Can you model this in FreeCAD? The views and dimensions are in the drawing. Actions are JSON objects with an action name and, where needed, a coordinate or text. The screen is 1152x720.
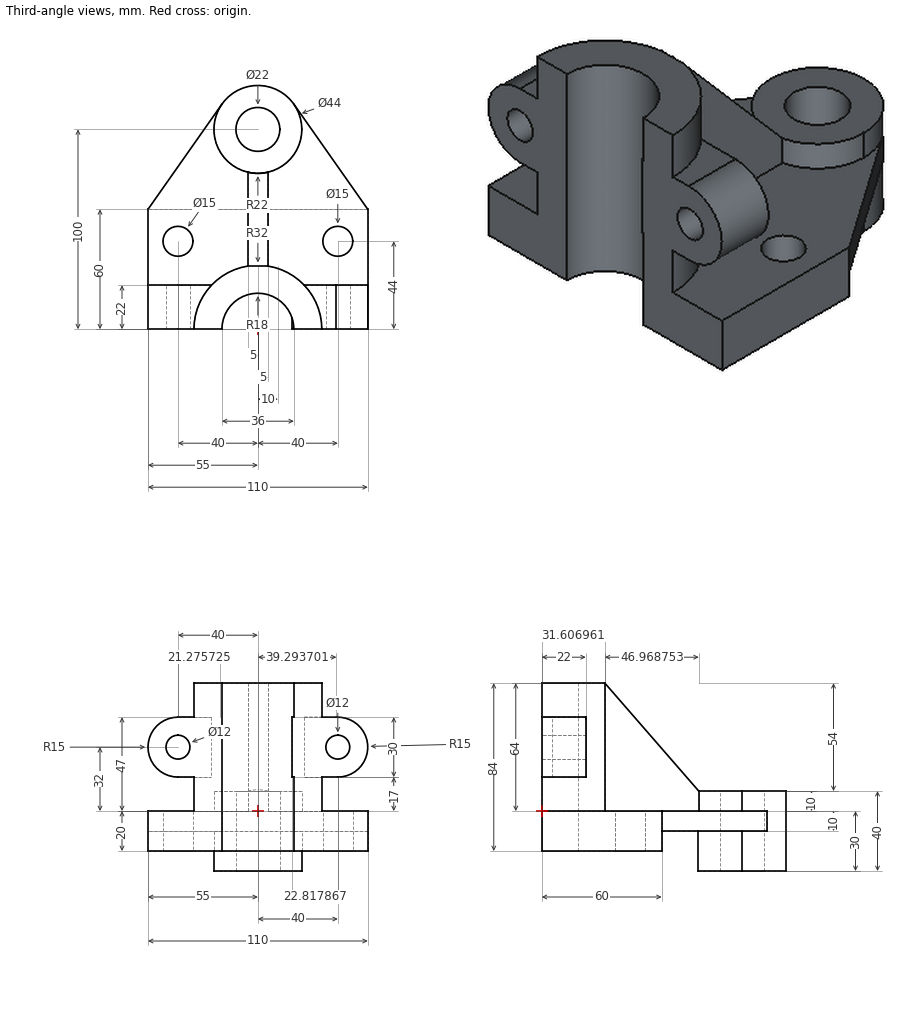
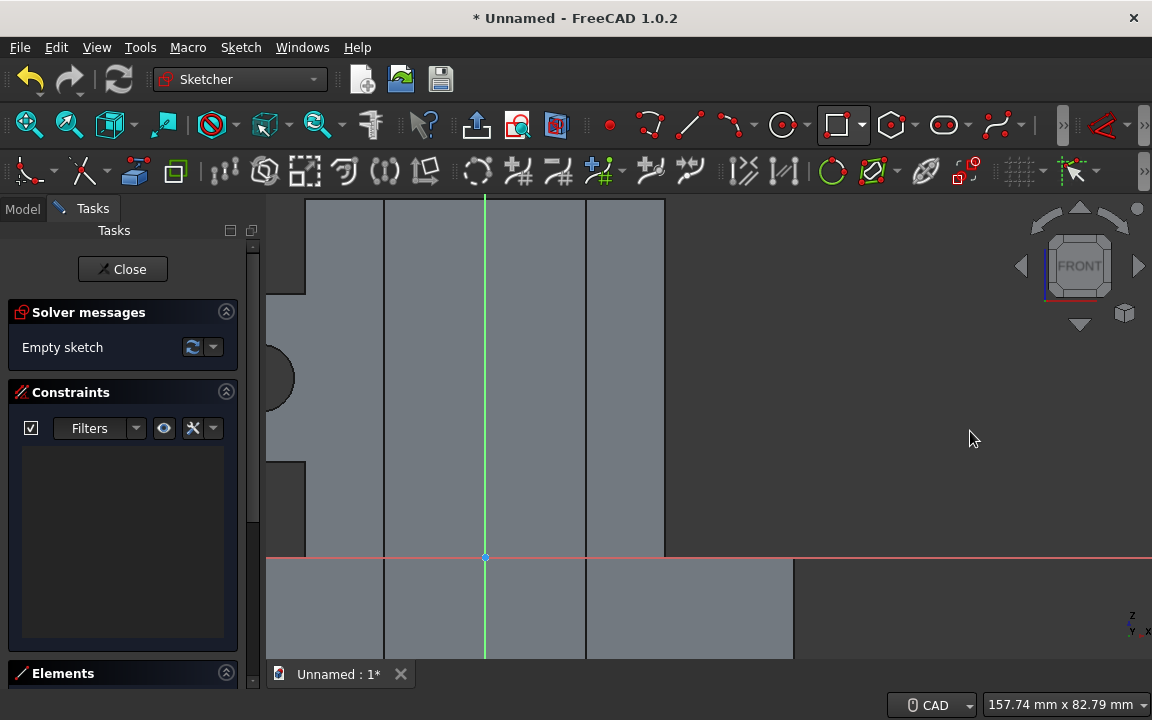
{"action": "left_click", "coordinate": [650, 126]}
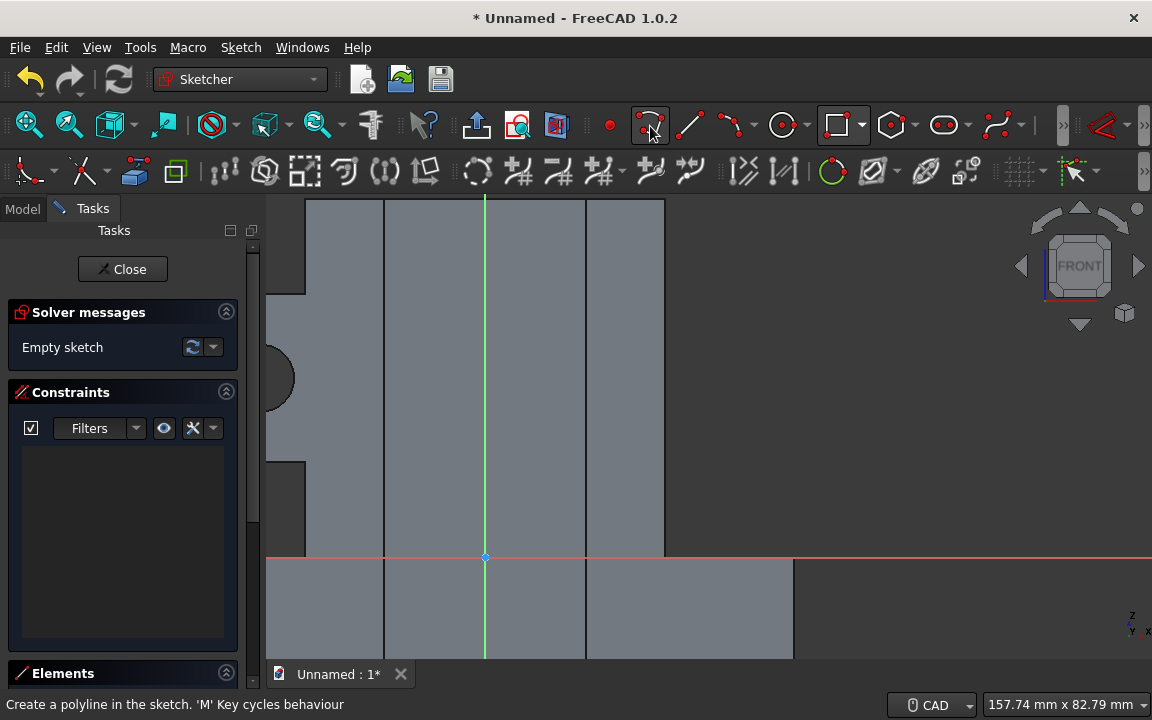
{"action": "left_click", "coordinate": [710, 462]}
{"action": "left_click", "coordinate": [582, 462]}
{"action": "left_click", "coordinate": [582, 294]}
{"action": "left_click", "coordinate": [706, 301]}
{"action": "right_click", "coordinate": [706, 301]}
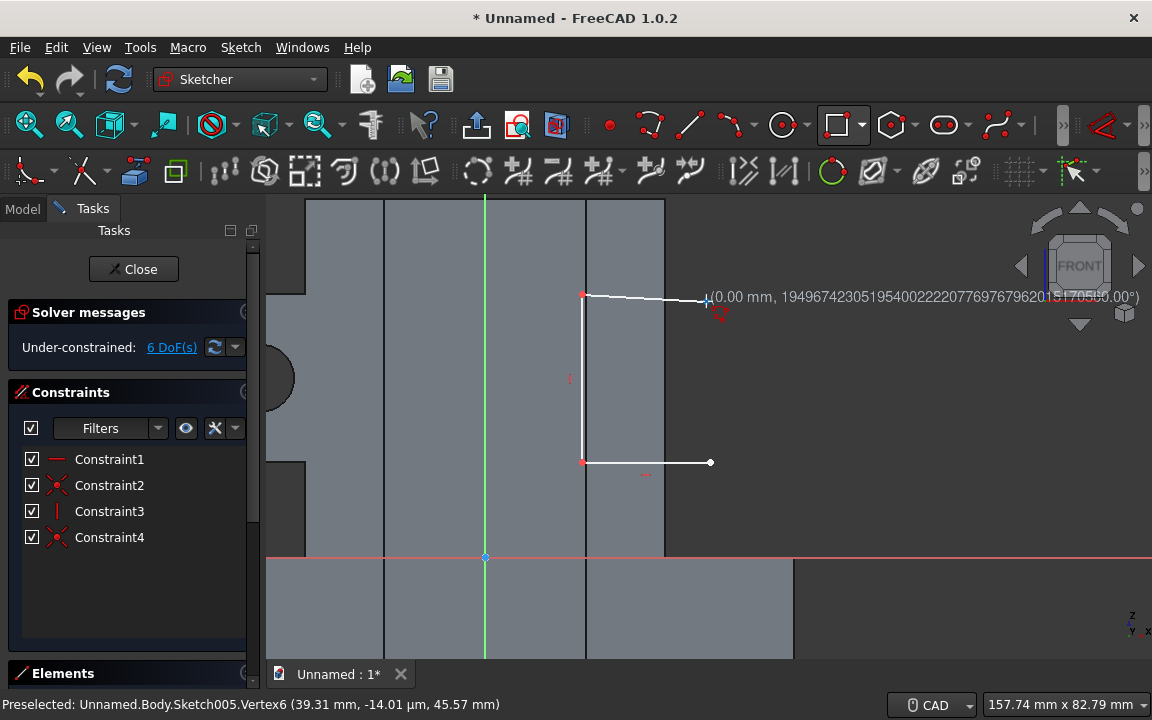
{"action": "left_click", "coordinate": [730, 126]}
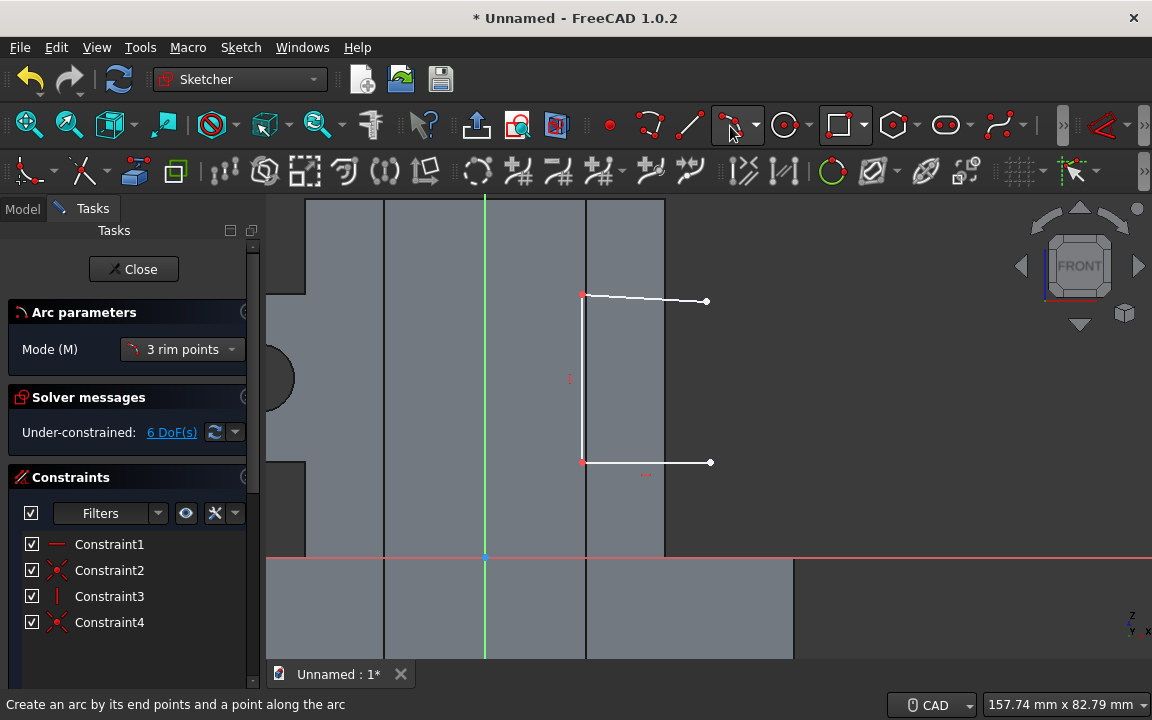
{"action": "left_click", "coordinate": [706, 302]}
{"action": "left_click", "coordinate": [710, 463]}
{"action": "left_click", "coordinate": [794, 376]}
{"action": "key", "text": "Escape"}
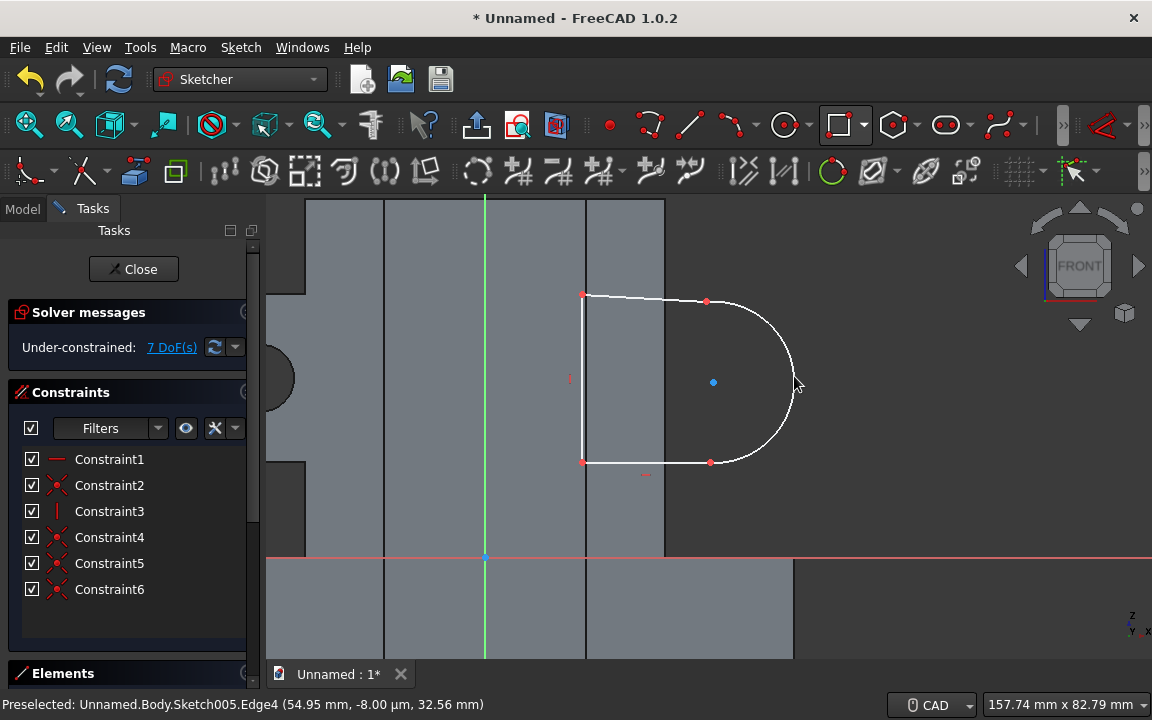
{"action": "left_click", "coordinate": [672, 463]}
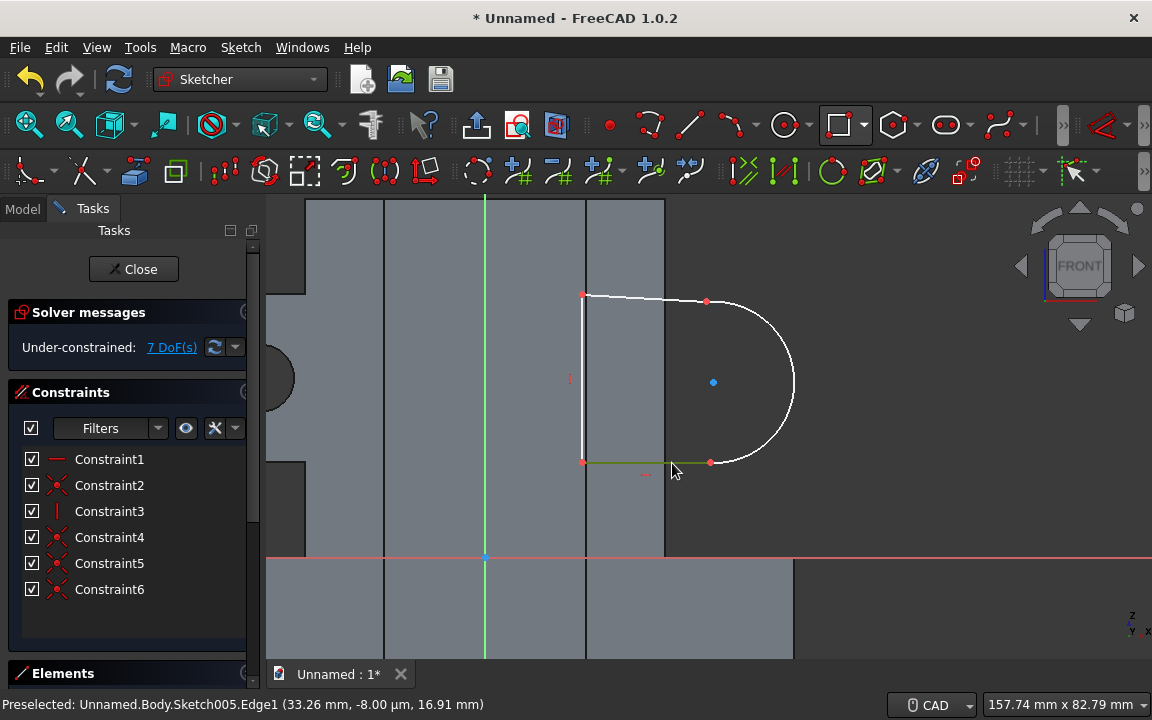
{"action": "left_click", "coordinate": [779, 430]}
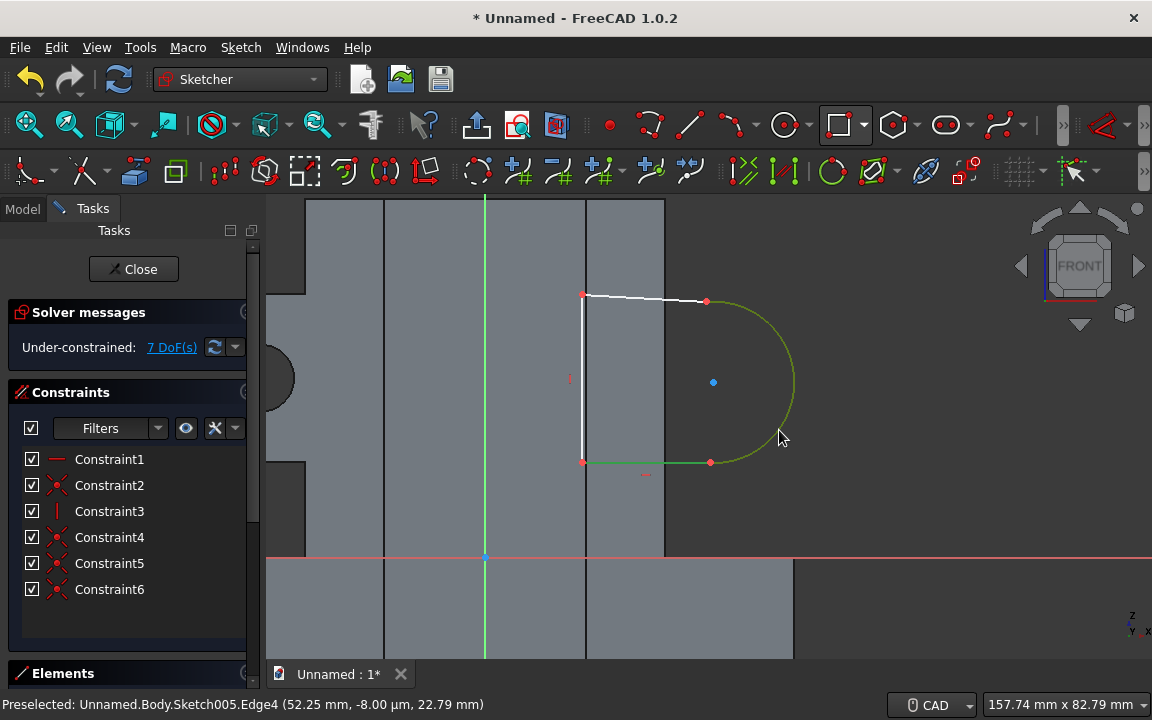
{"action": "key", "text": "t"}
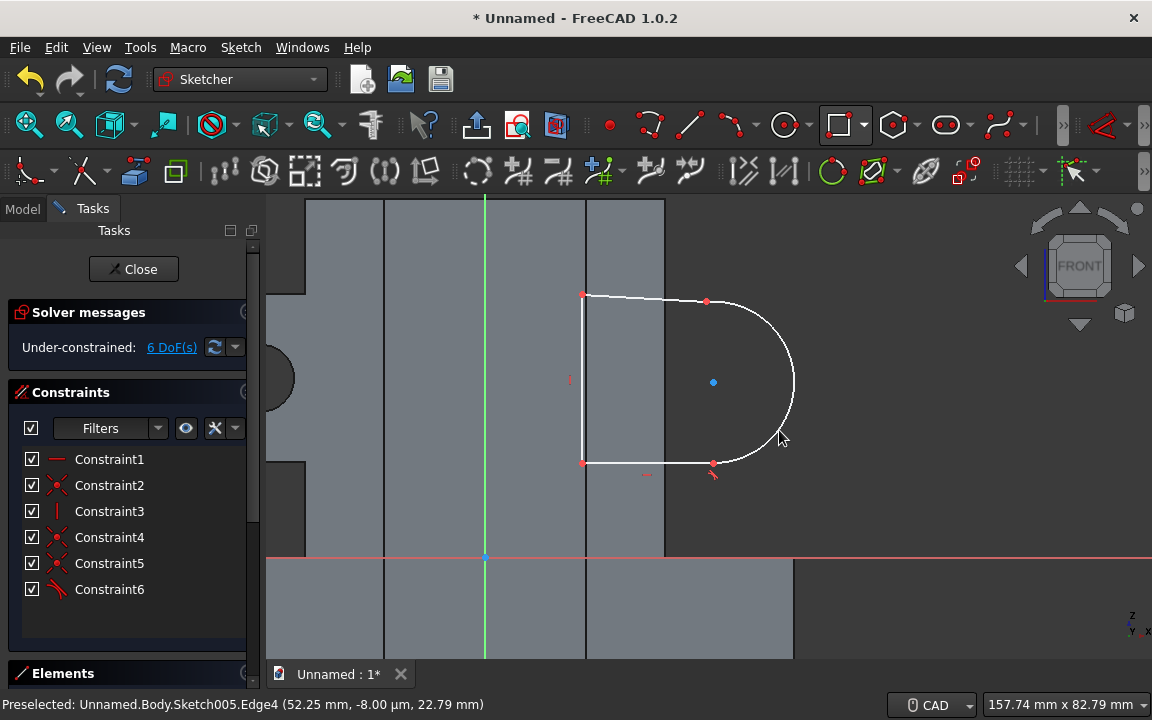
{"action": "left_click", "coordinate": [1102, 126]}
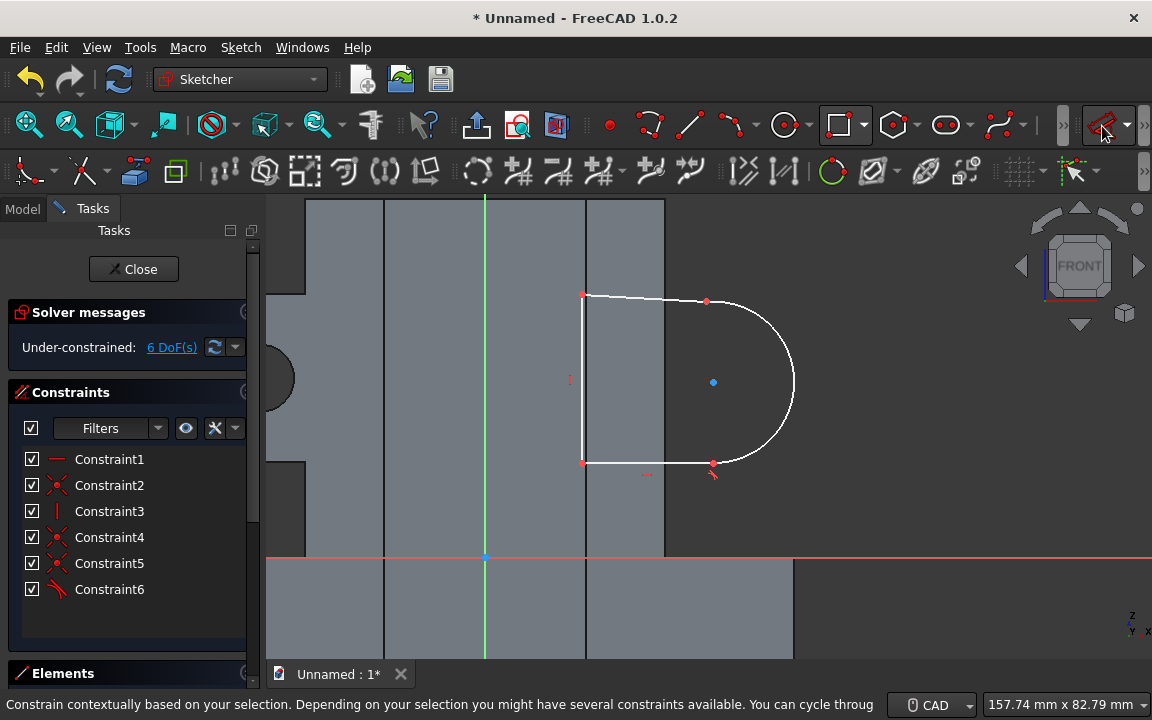
{"action": "left_click", "coordinate": [780, 428]}
{"action": "left_click", "coordinate": [806, 446]}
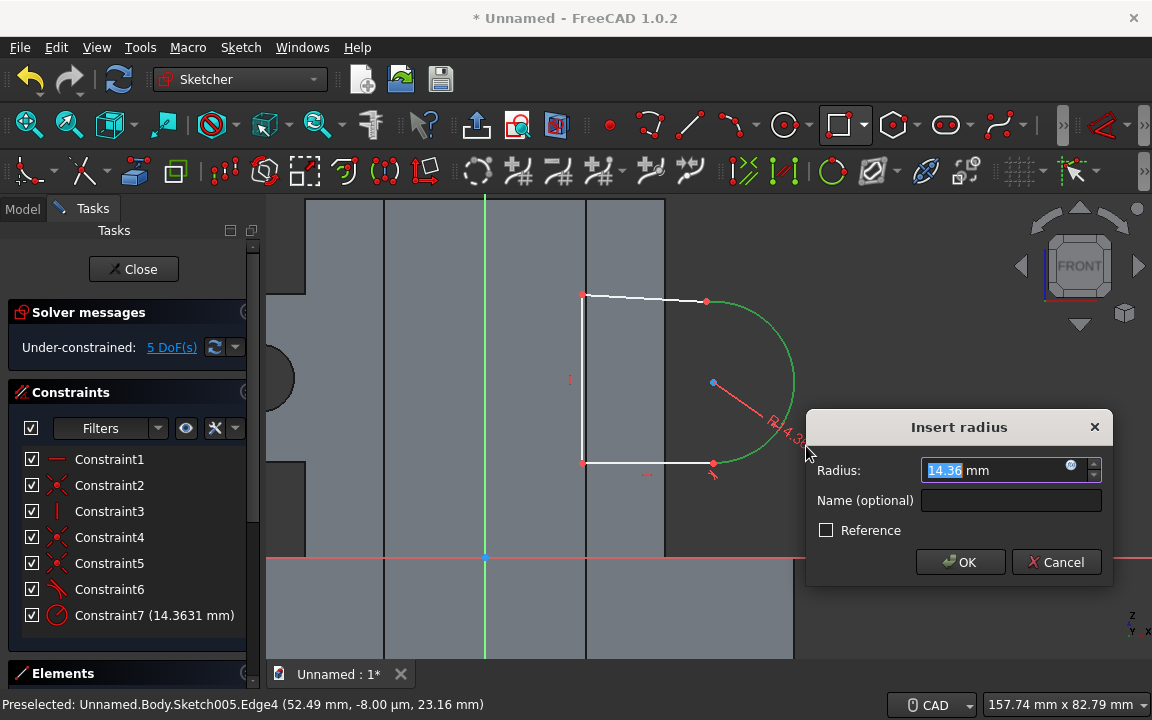
{"action": "type", "text": "15"}
{"action": "key", "text": "Return"}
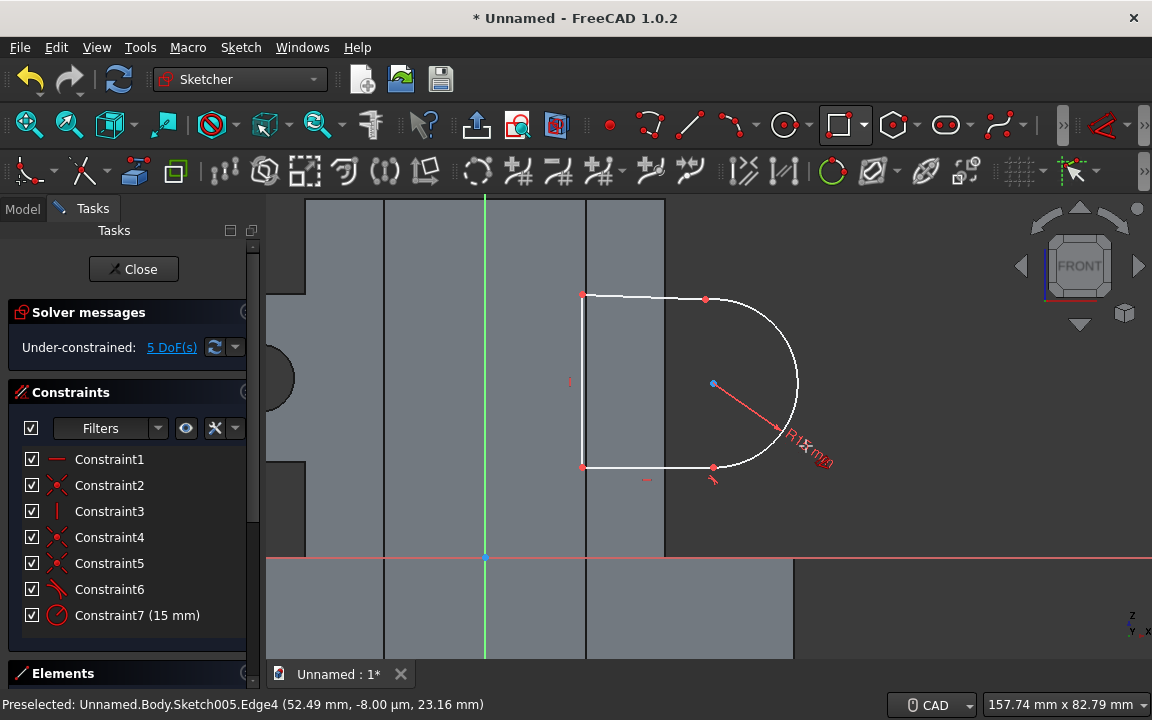
{"action": "left_click", "coordinate": [582, 416]}
{"action": "left_click", "coordinate": [548, 381]}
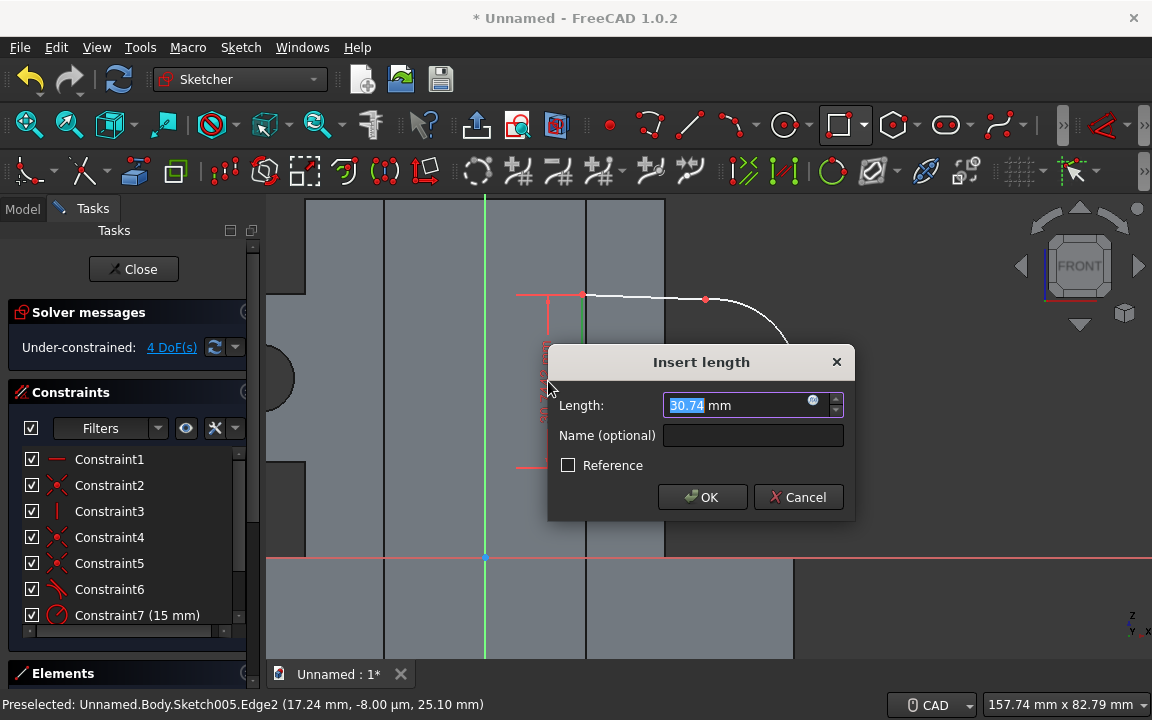
{"action": "type", "text": "30"}
{"action": "key", "text": "Return"}